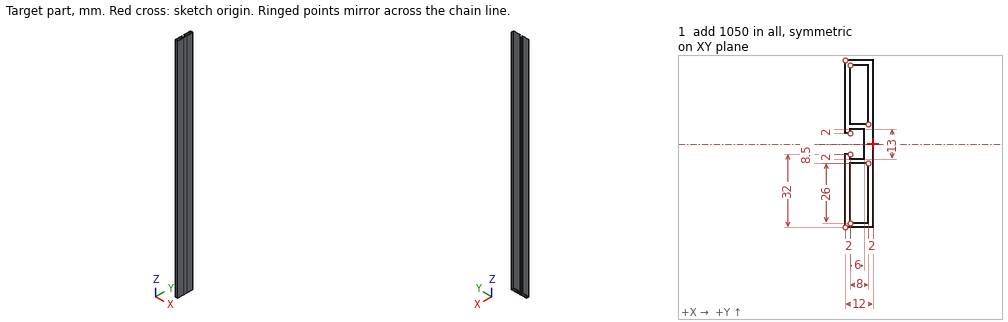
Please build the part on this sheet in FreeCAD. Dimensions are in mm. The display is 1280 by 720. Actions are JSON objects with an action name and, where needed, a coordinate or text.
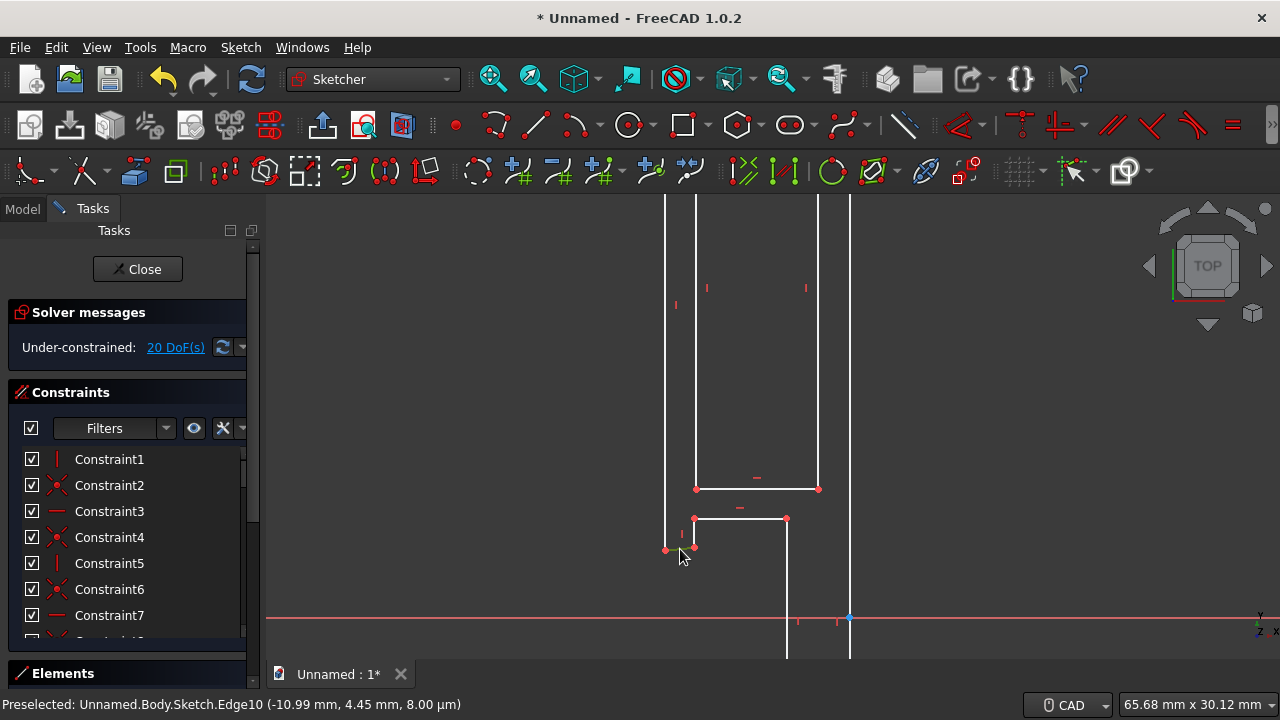
{"action": "key", "text": "h"}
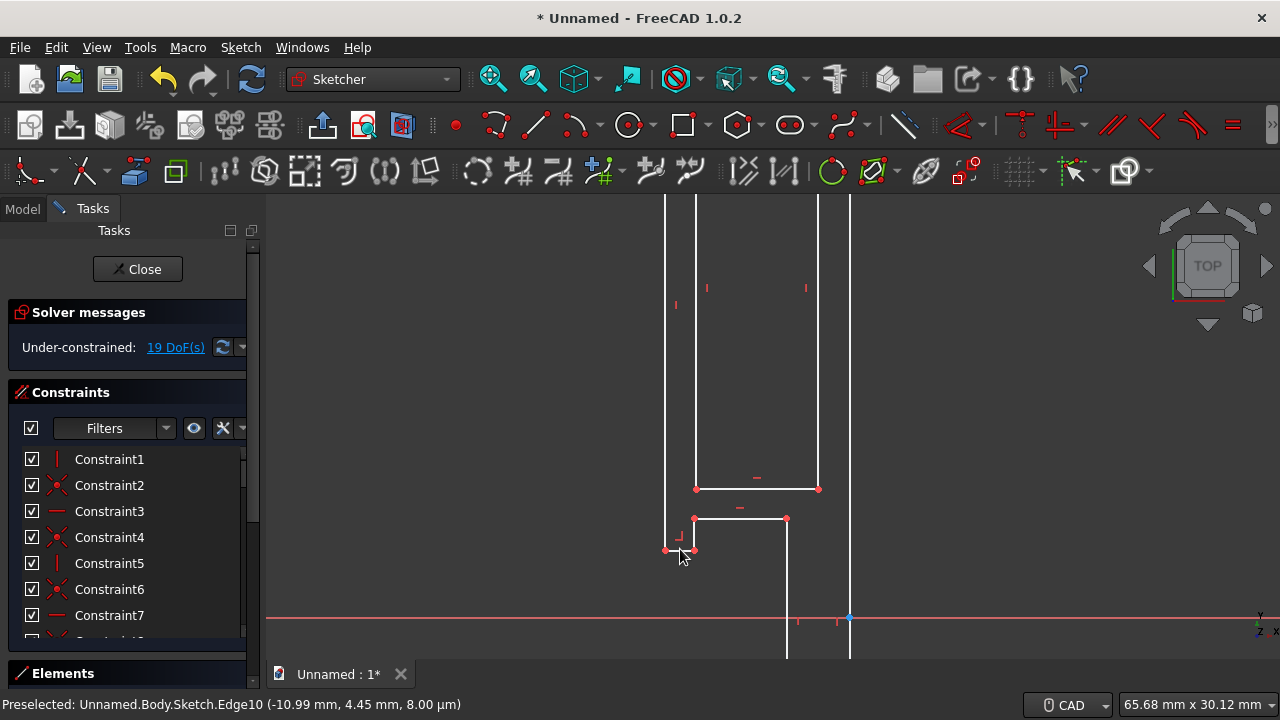
{"action": "scroll", "coordinate": [687, 364], "scroll_direction": "down", "scroll_amount": 7}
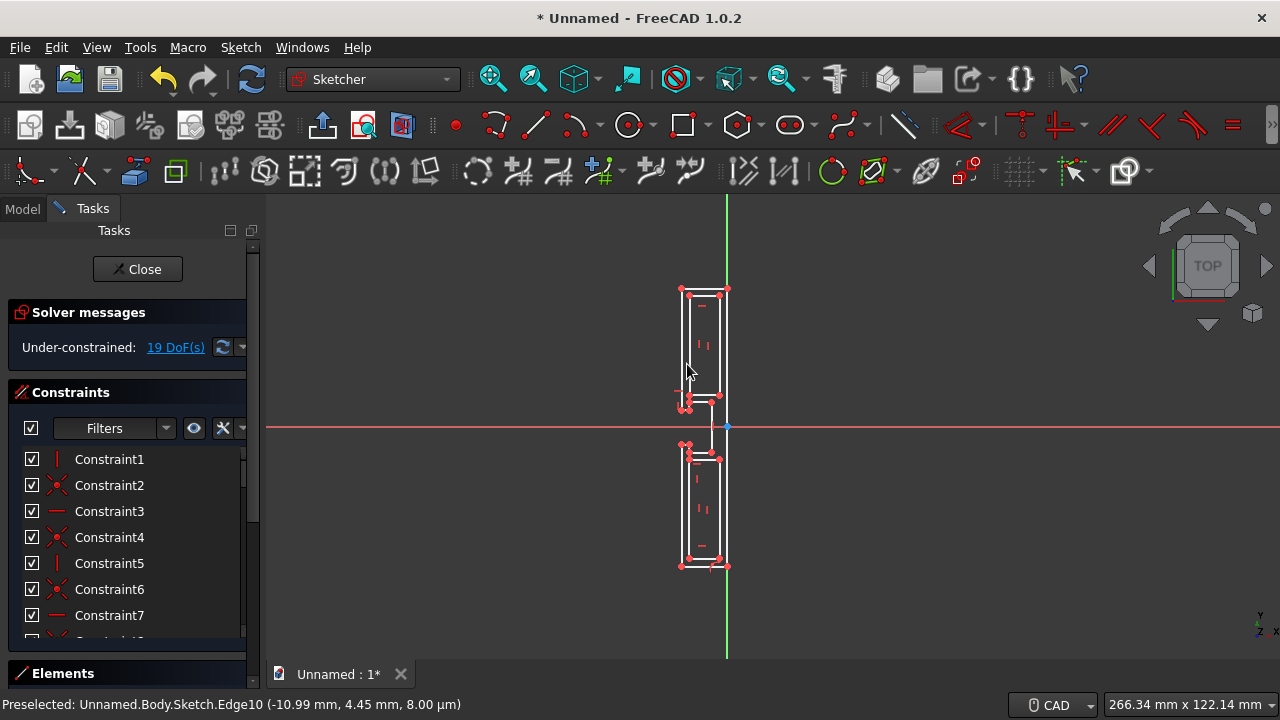
{"action": "left_click", "coordinate": [682, 567]}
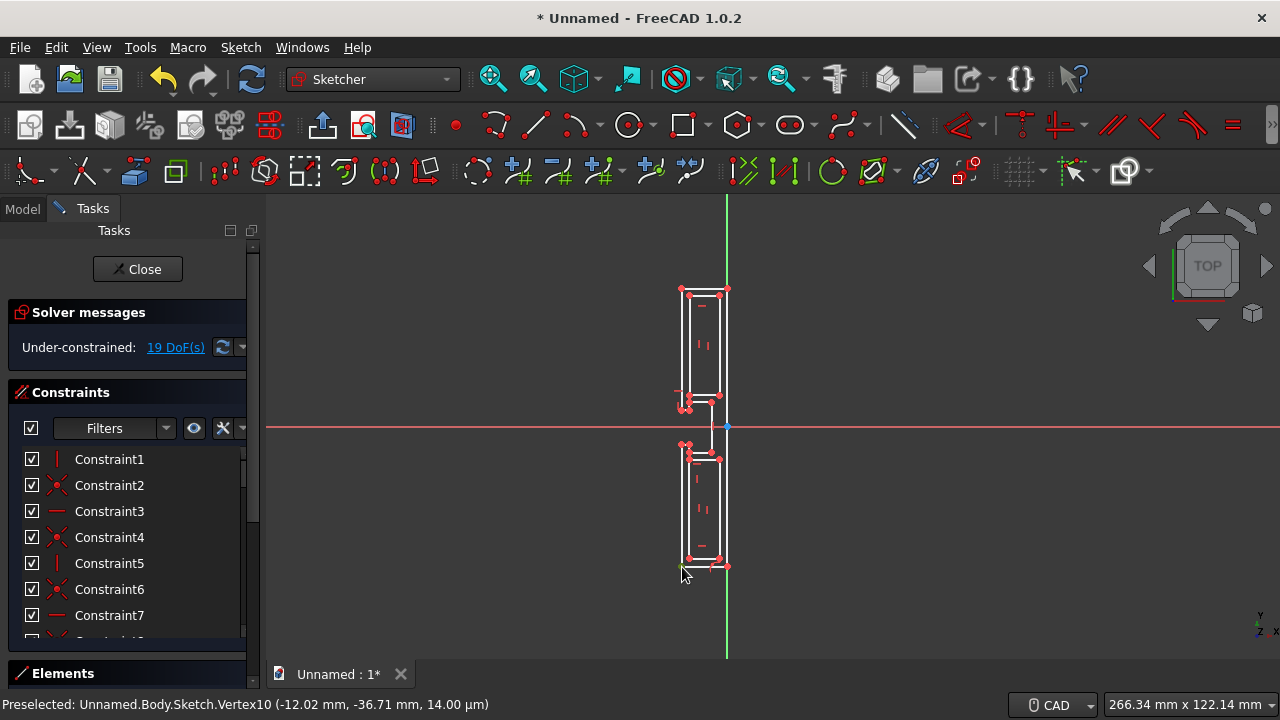
{"action": "left_click", "coordinate": [682, 289]}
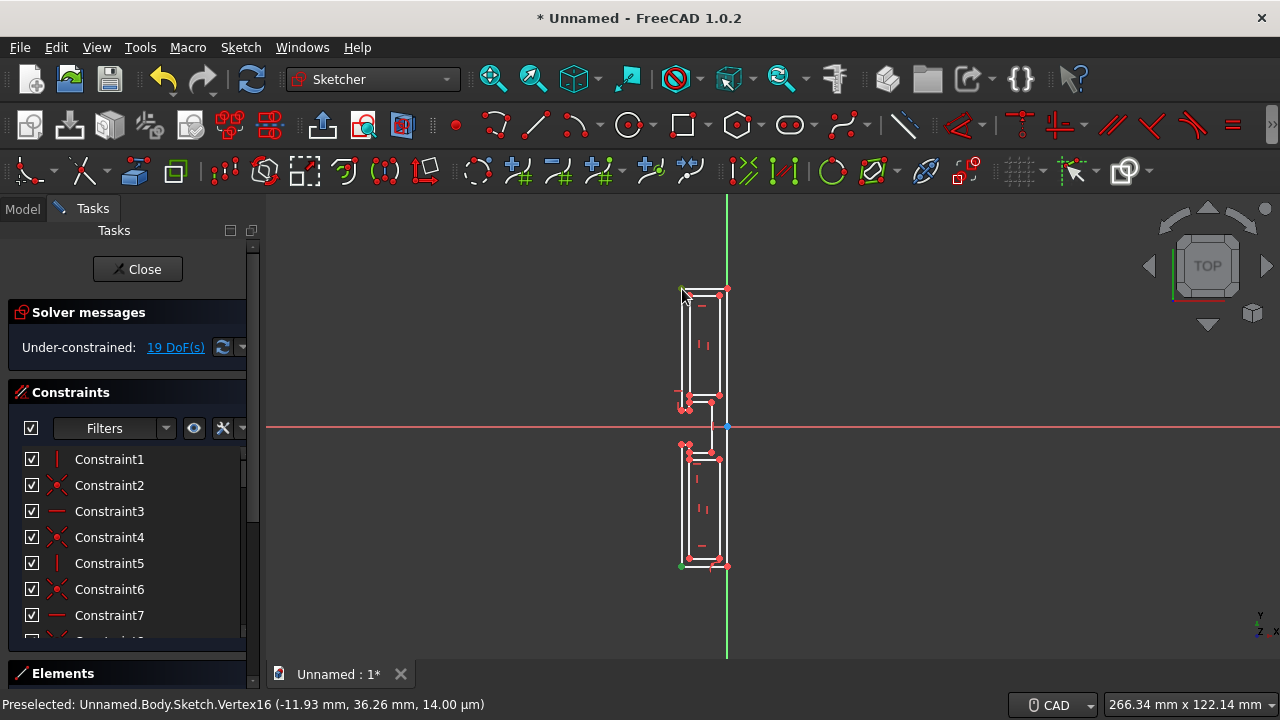
{"action": "left_click", "coordinate": [353, 427]}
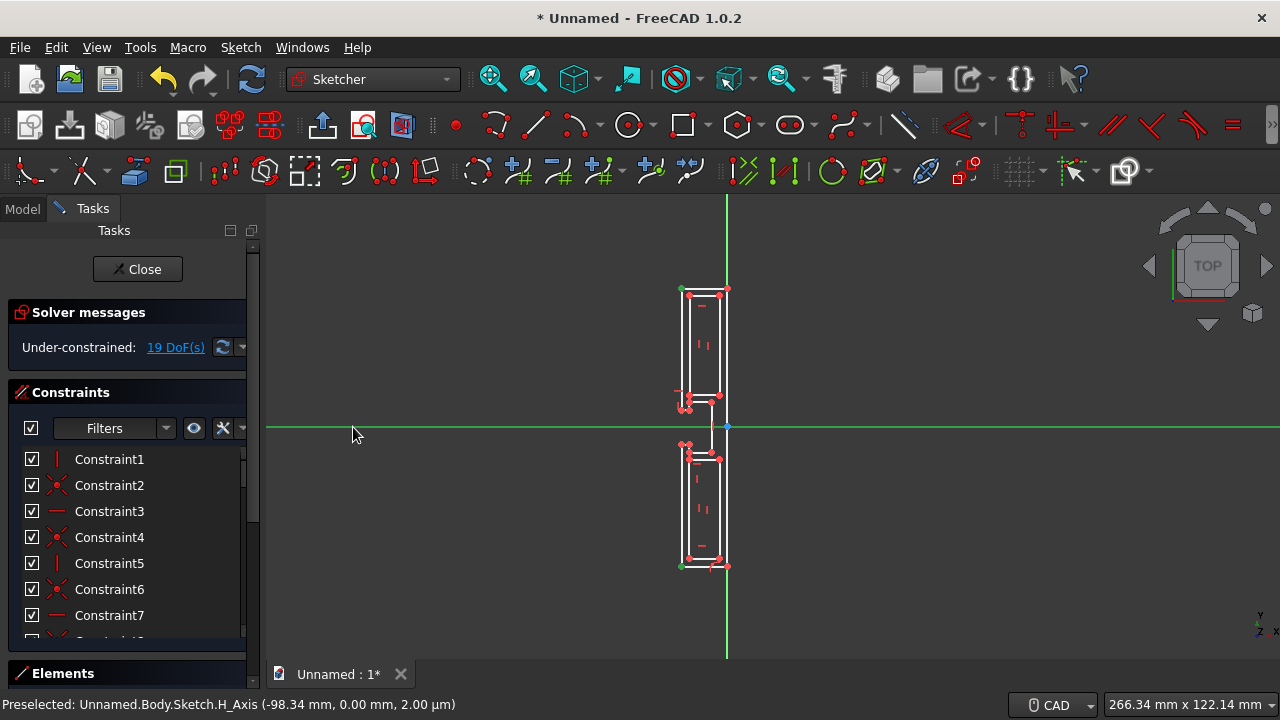
{"action": "key", "text": "s"}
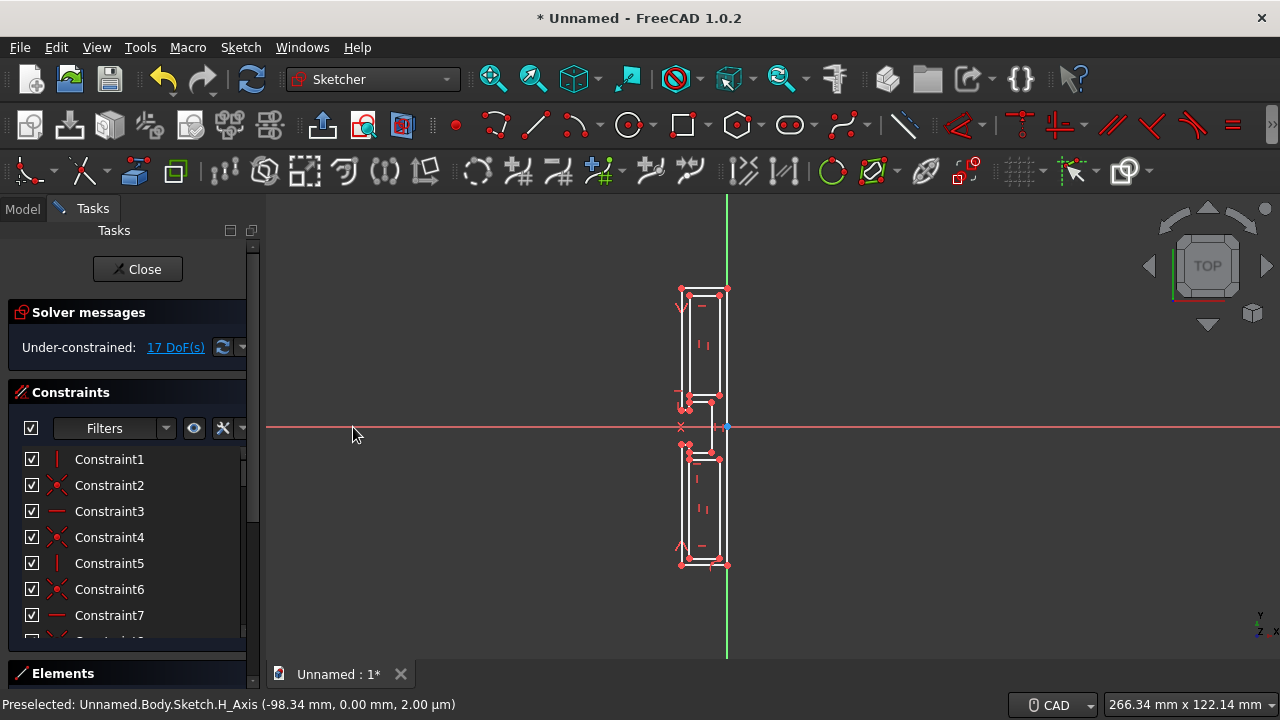
{"action": "scroll", "coordinate": [689, 445], "scroll_direction": "up", "scroll_amount": 3}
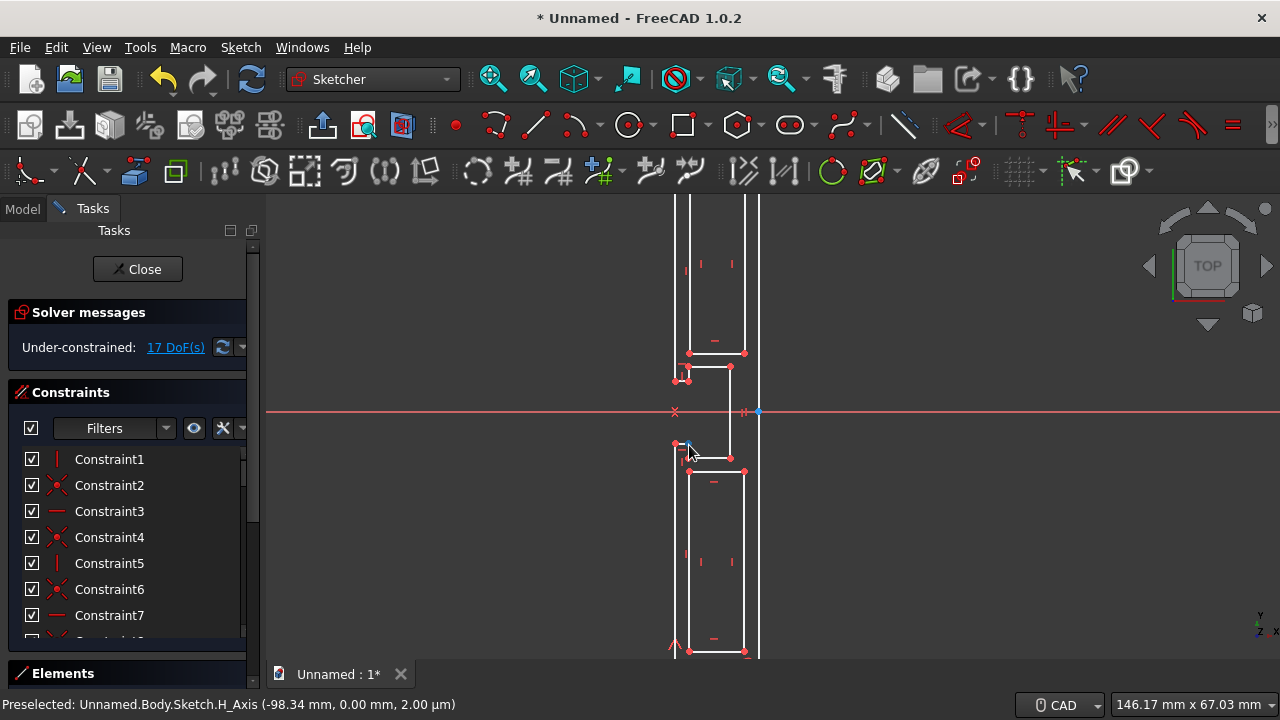
{"action": "left_click", "coordinate": [689, 444]}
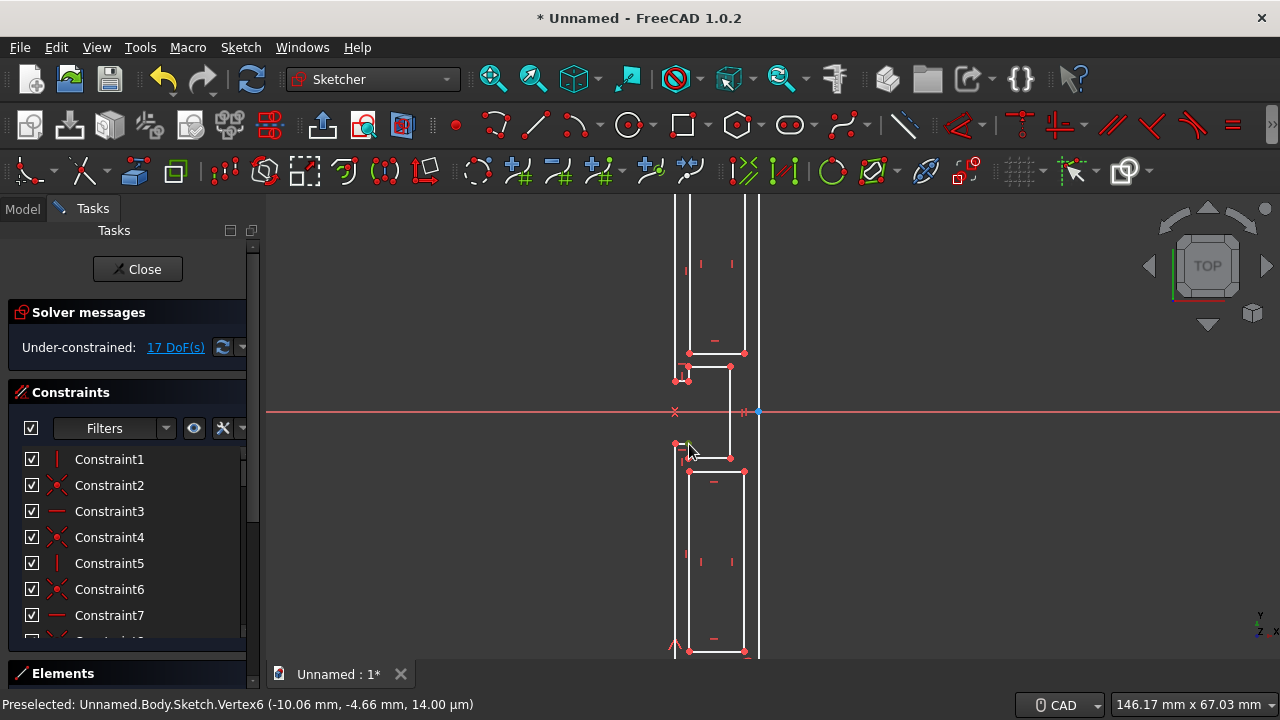
{"action": "left_click", "coordinate": [689, 381]}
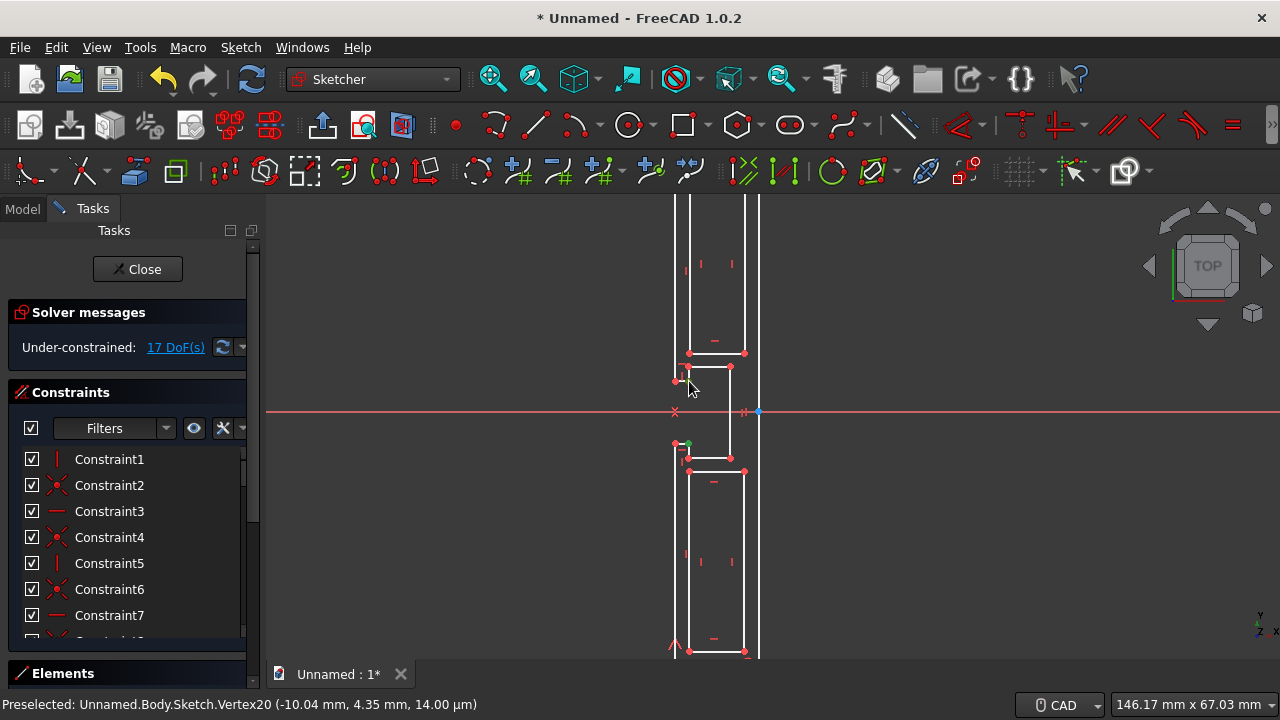
{"action": "left_click", "coordinate": [353, 412]}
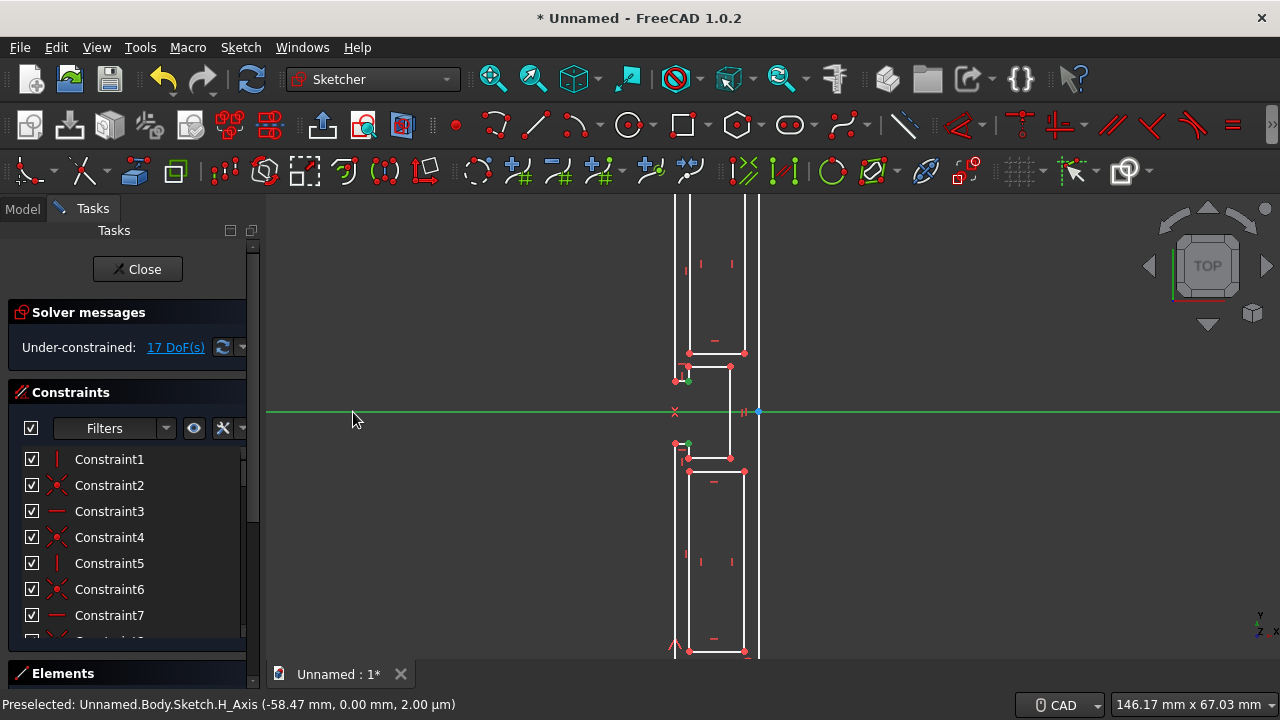
{"action": "key", "text": "s"}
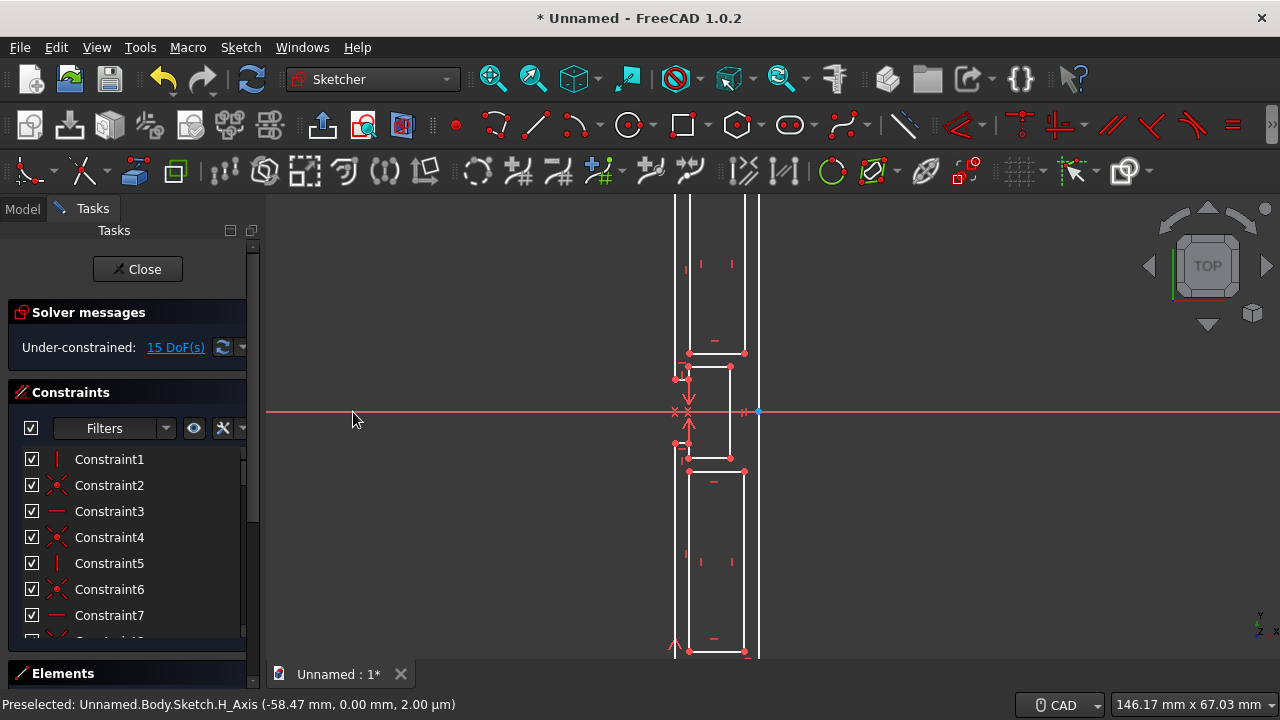
{"action": "scroll", "coordinate": [689, 445], "scroll_direction": "down", "scroll_amount": 3}